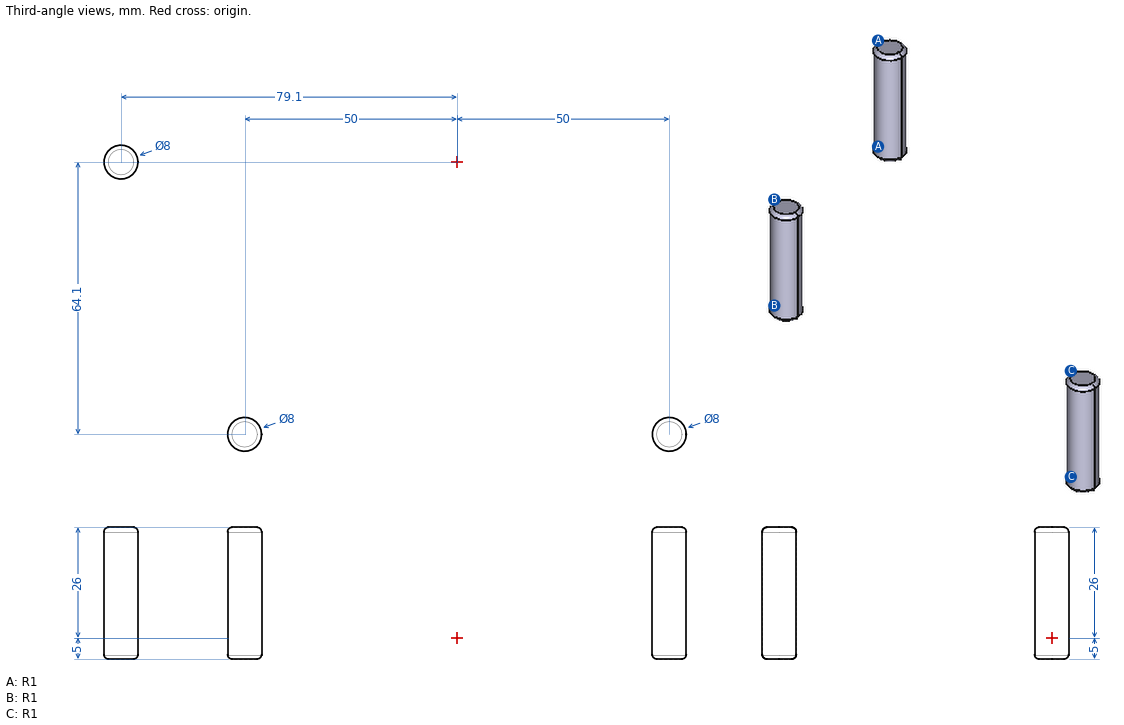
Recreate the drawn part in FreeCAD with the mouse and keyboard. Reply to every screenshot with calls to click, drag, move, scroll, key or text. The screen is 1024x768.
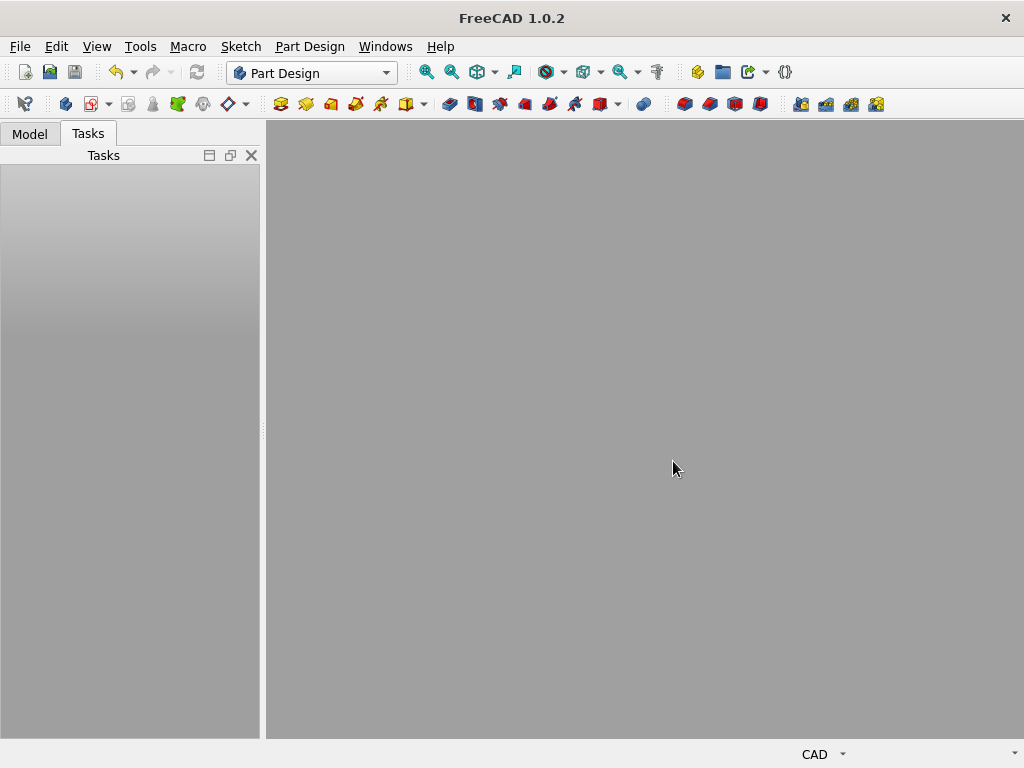
click(25, 72)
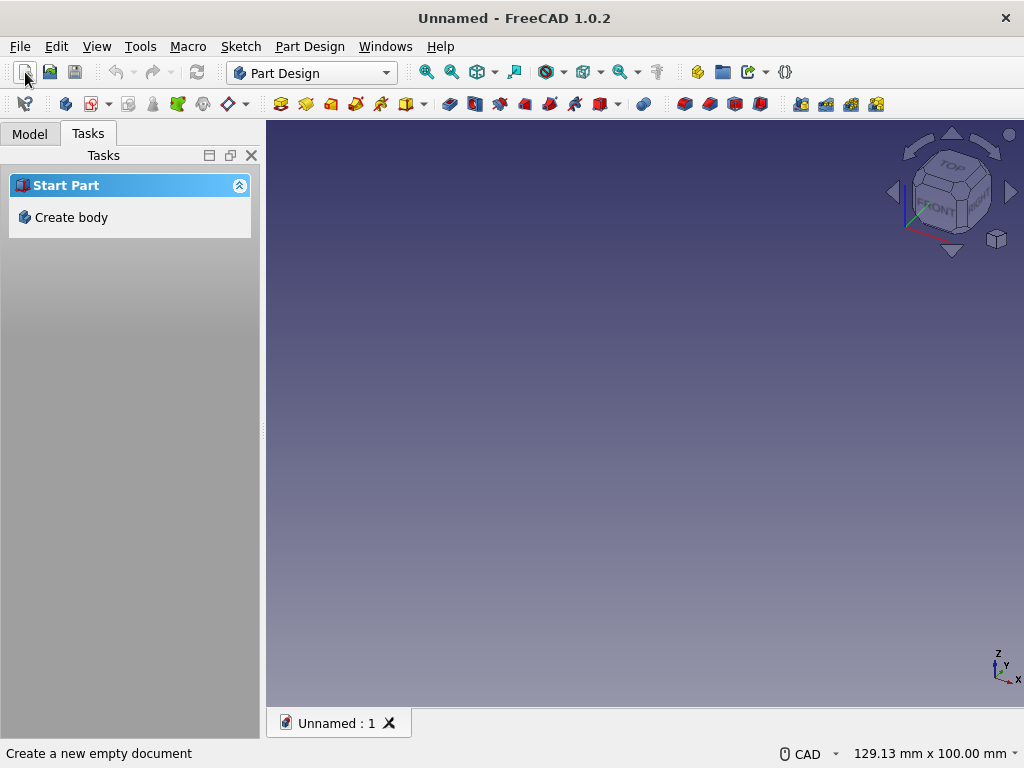
click(90, 104)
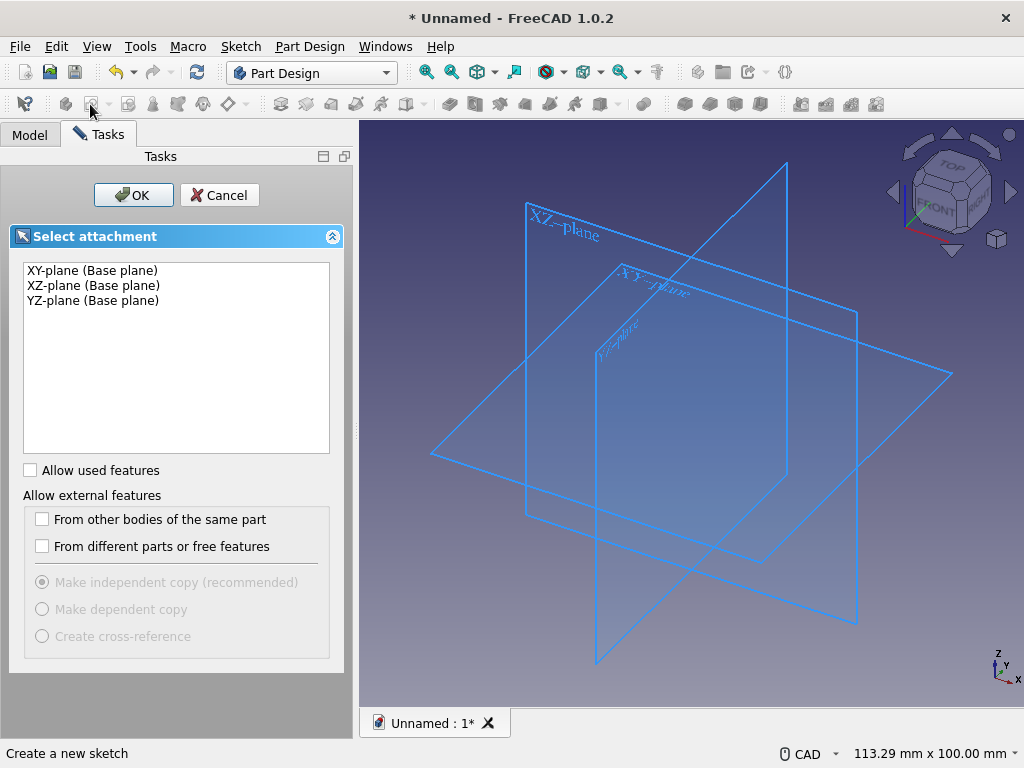
click(84, 270)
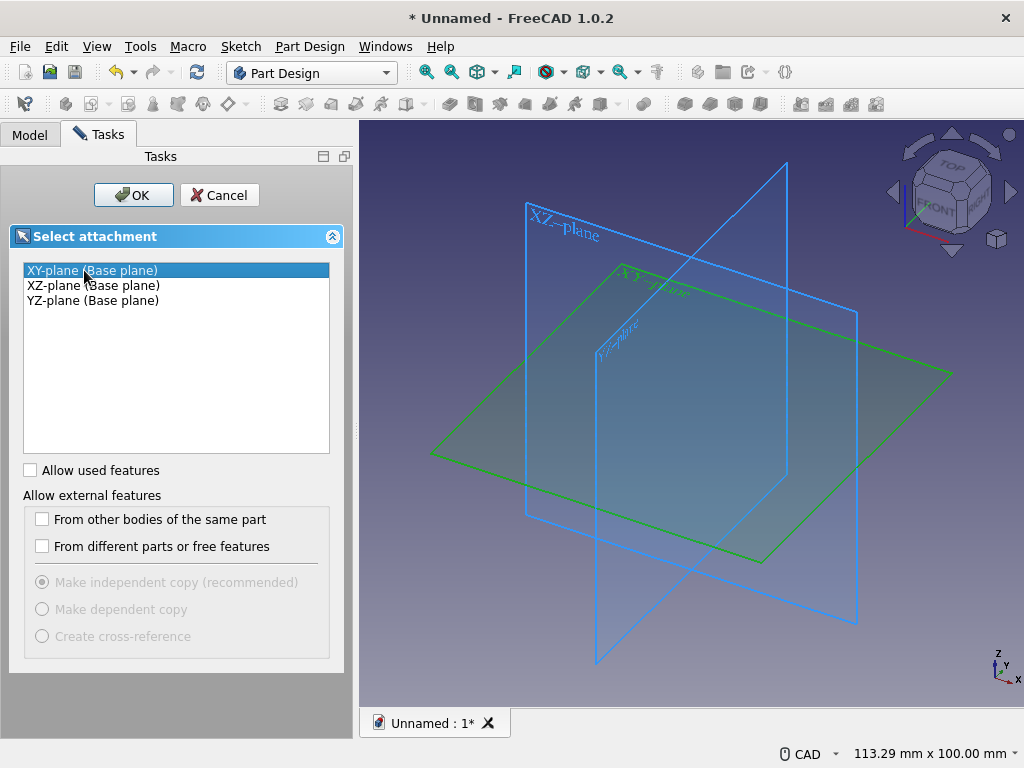
click(134, 195)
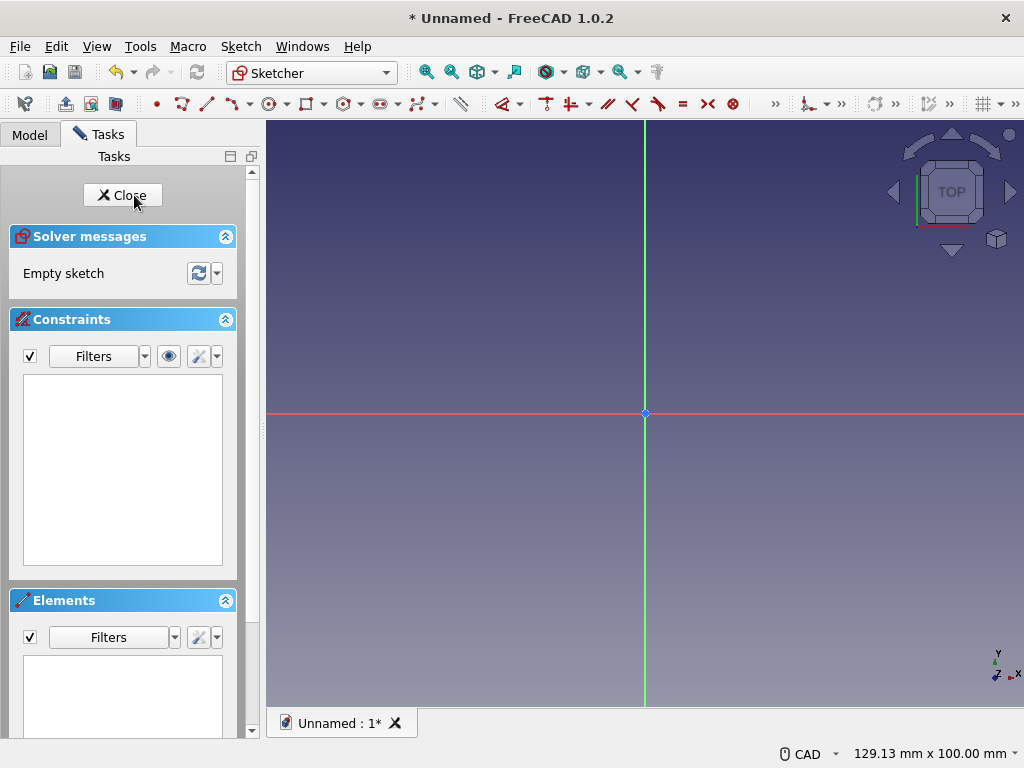
scroll(576, 414, down, 5)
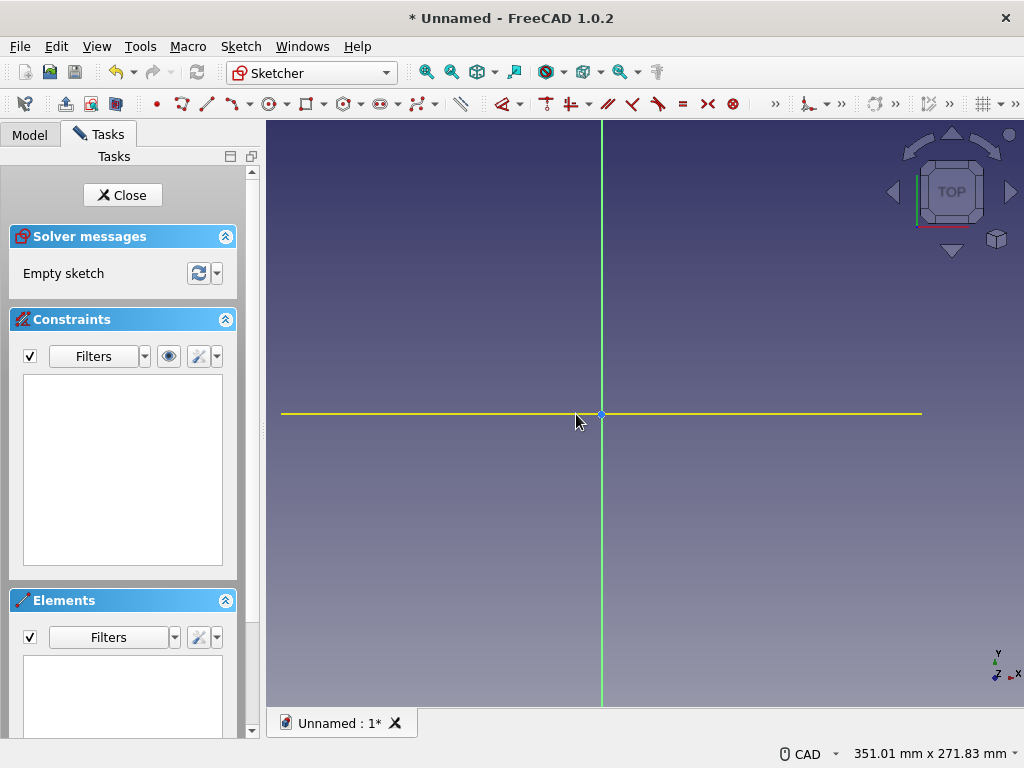
scroll(423, 414, up, 15)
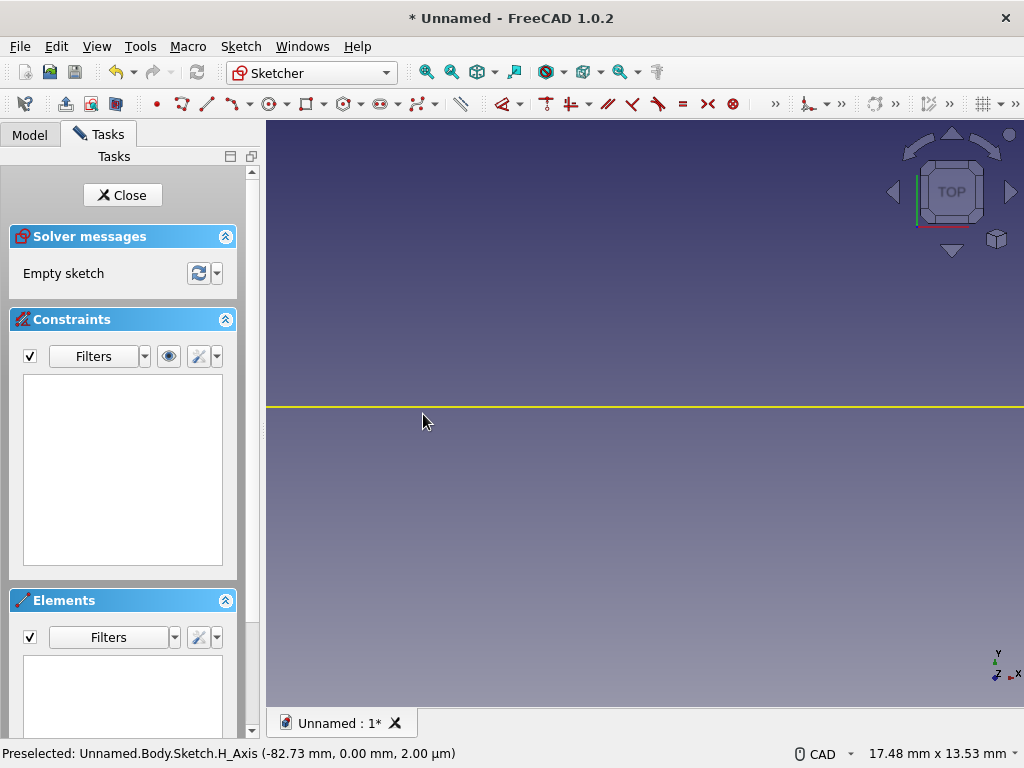
click(268, 104)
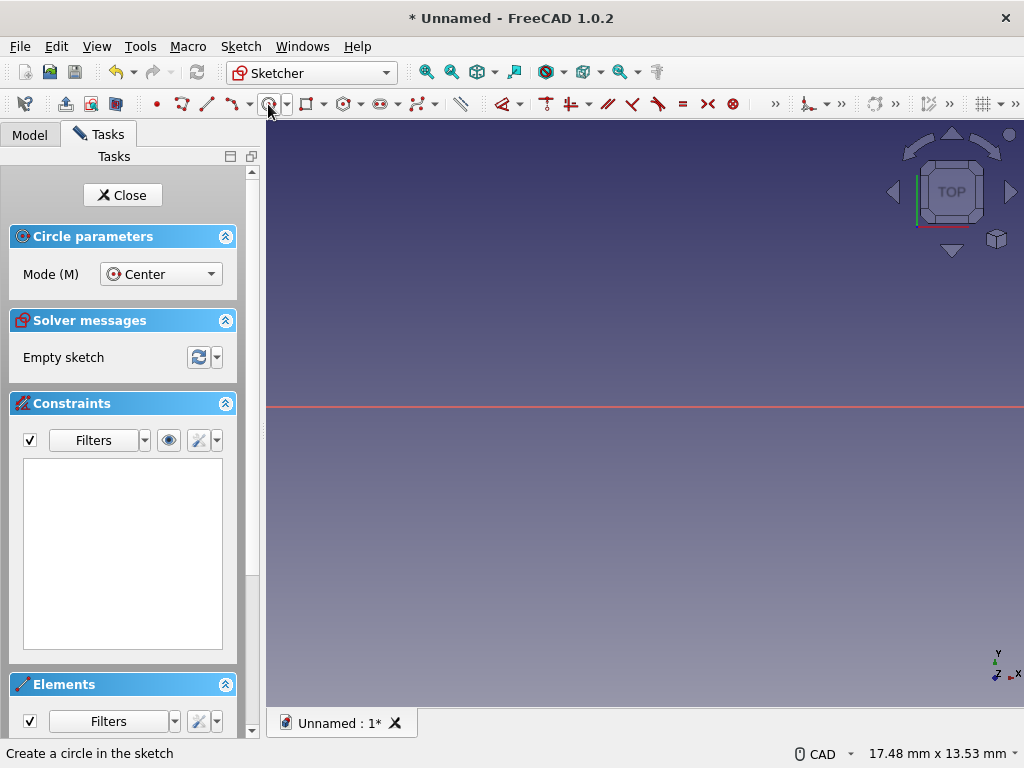
click(576, 407)
click(699, 284)
key(Escape)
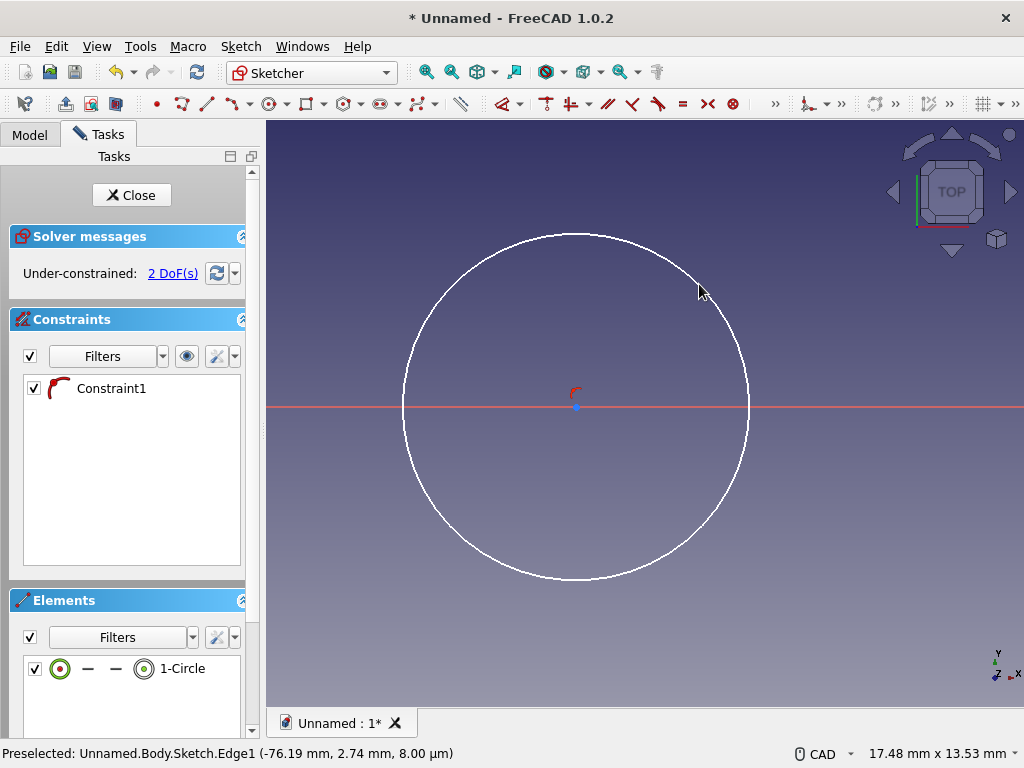
click(502, 104)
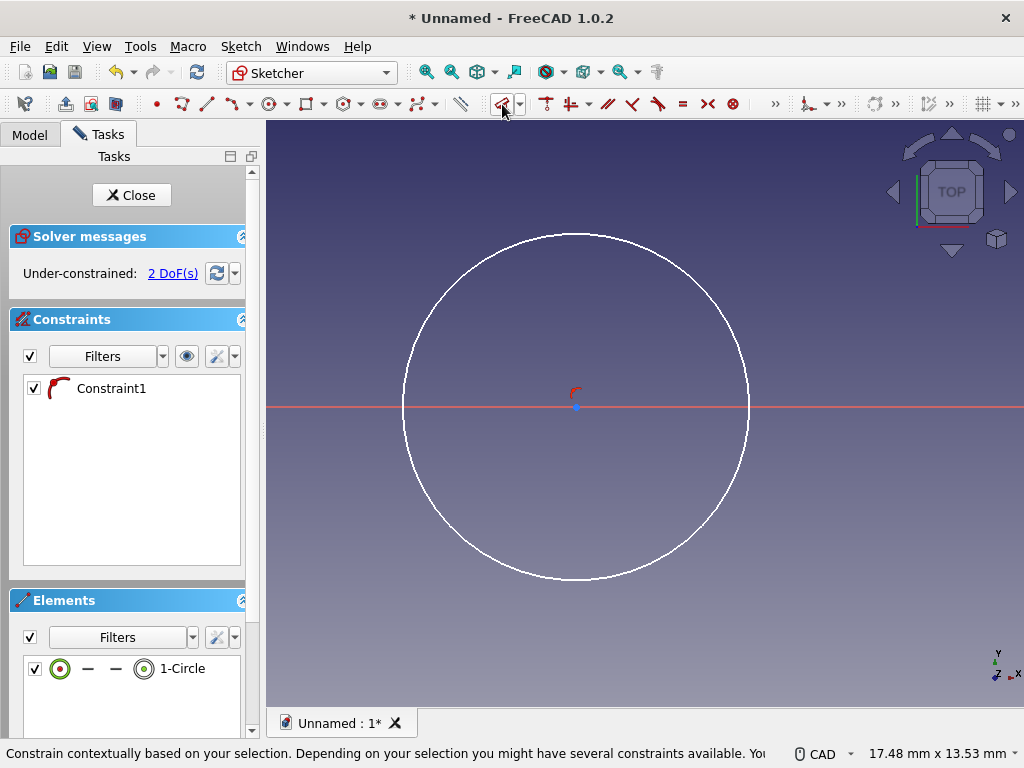
click(698, 284)
click(721, 261)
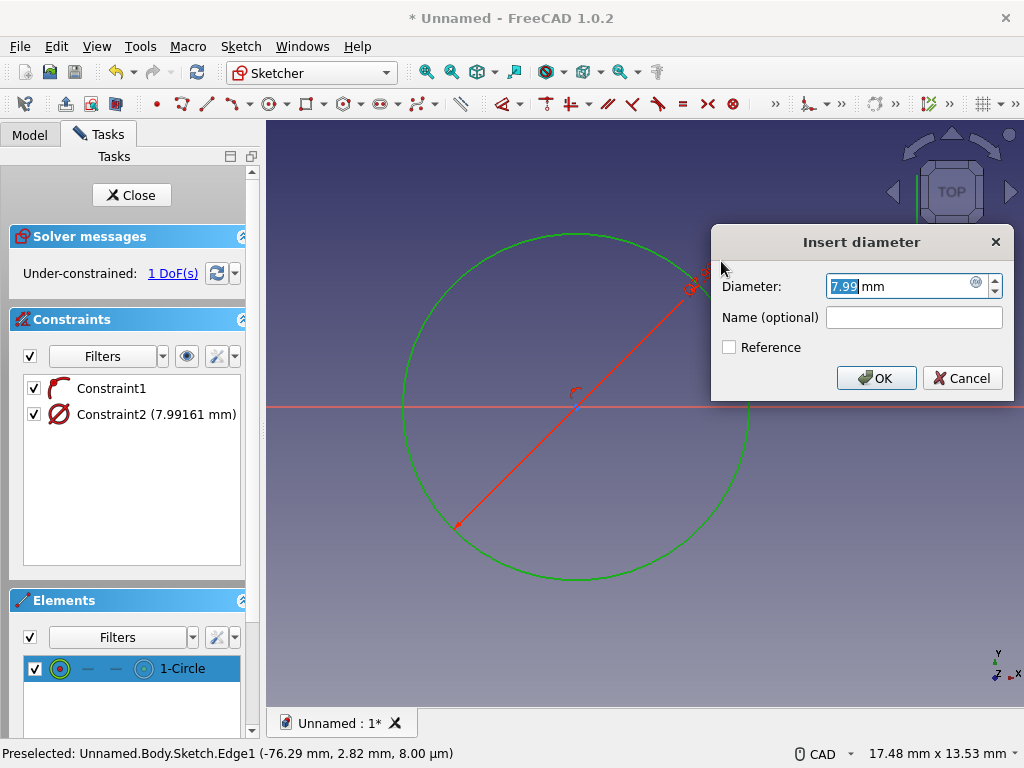
text(8)
key(Return)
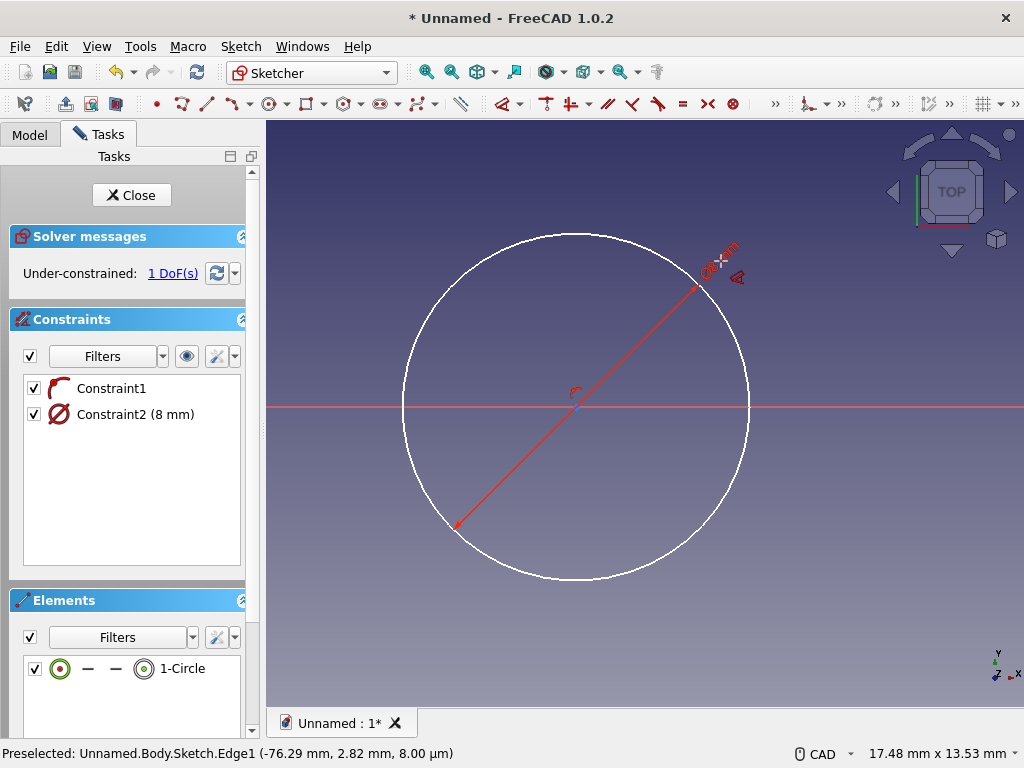
click(576, 407)
click(718, 441)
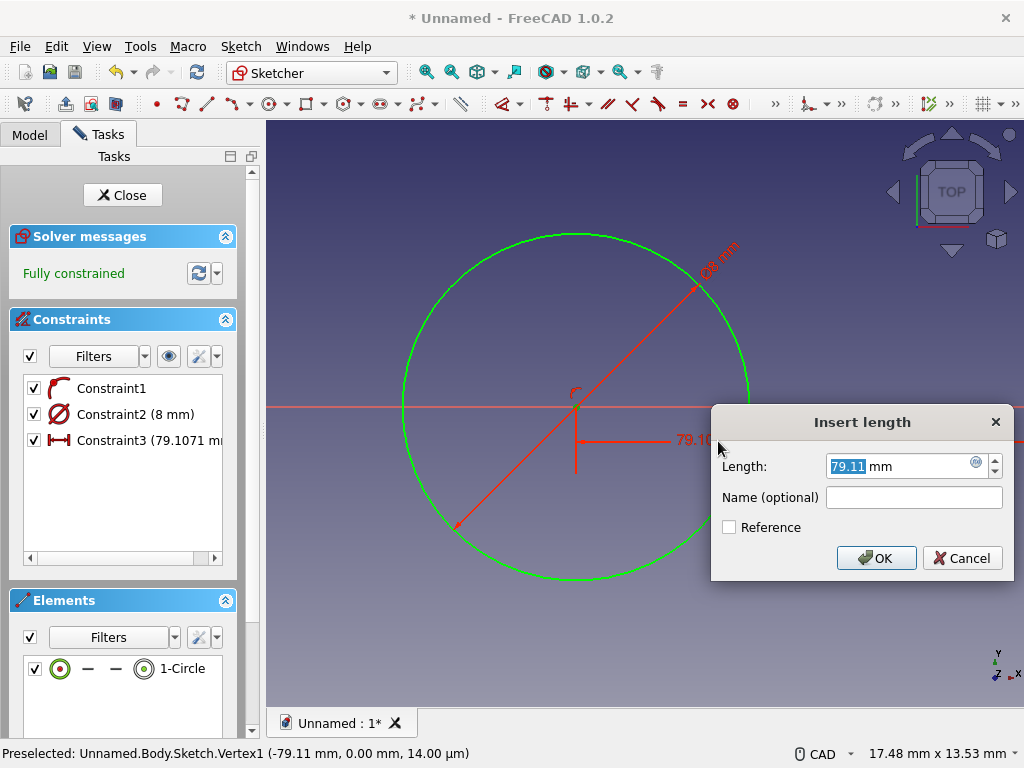
text(79.1)
key(Return)
key(Escape)